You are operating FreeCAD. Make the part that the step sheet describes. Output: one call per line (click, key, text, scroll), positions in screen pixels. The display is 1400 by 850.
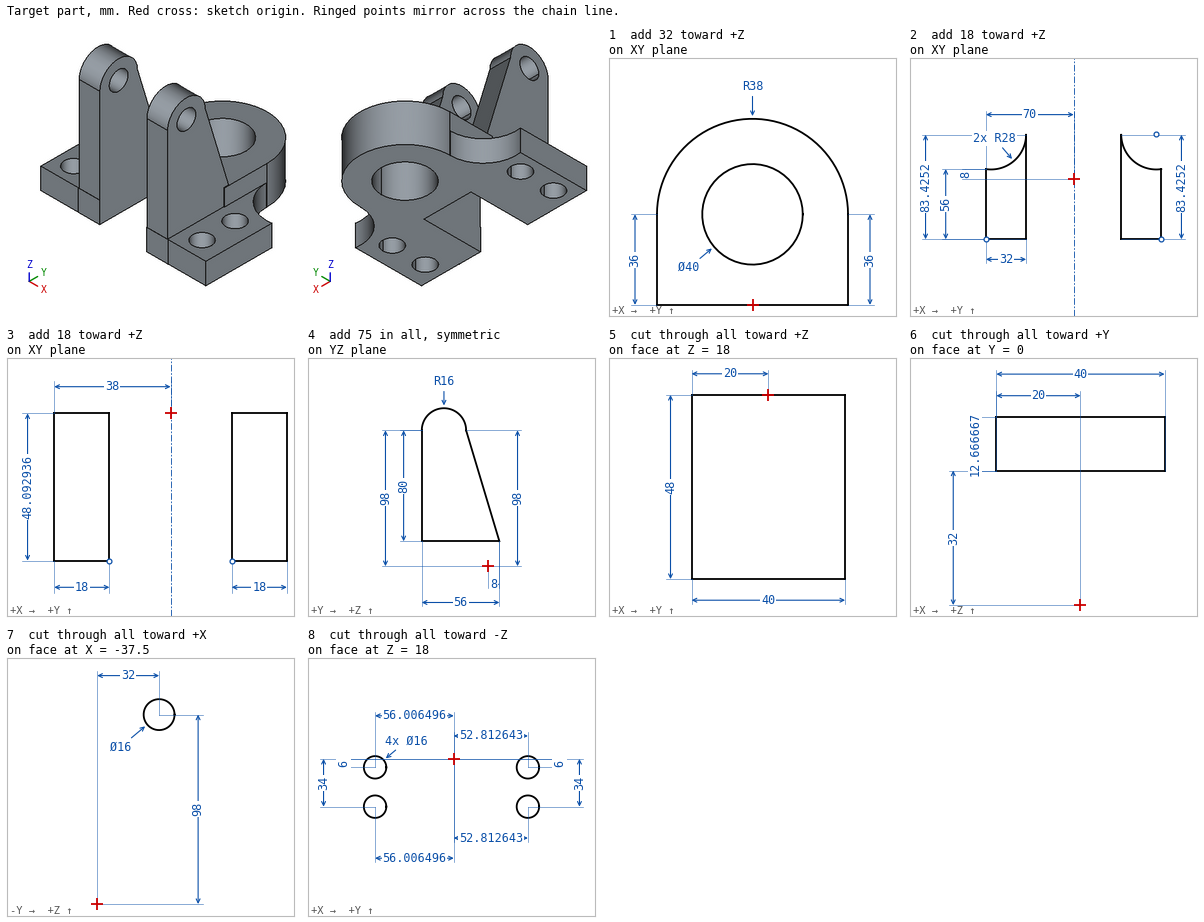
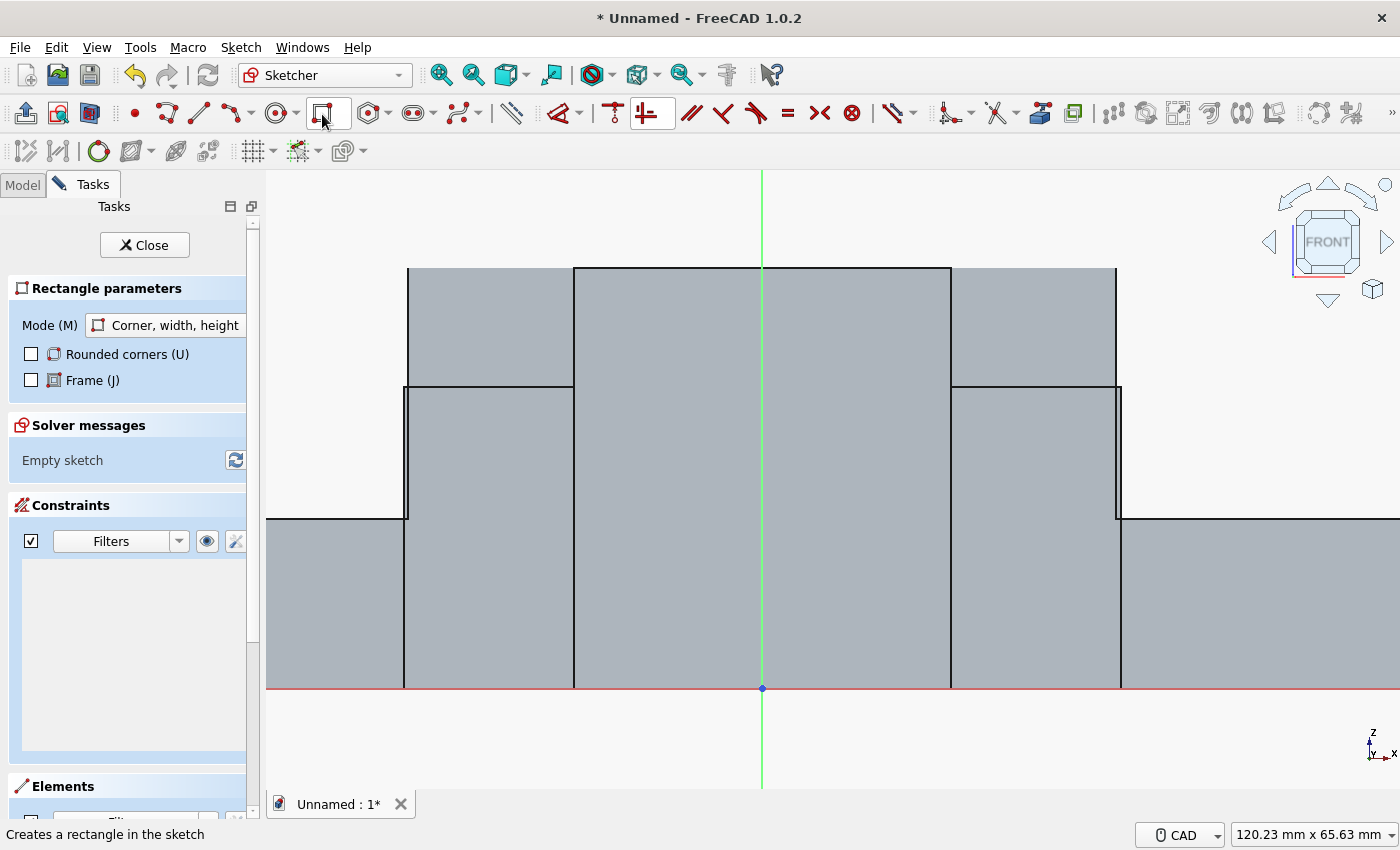
click(574, 268)
click(951, 387)
key(Escape)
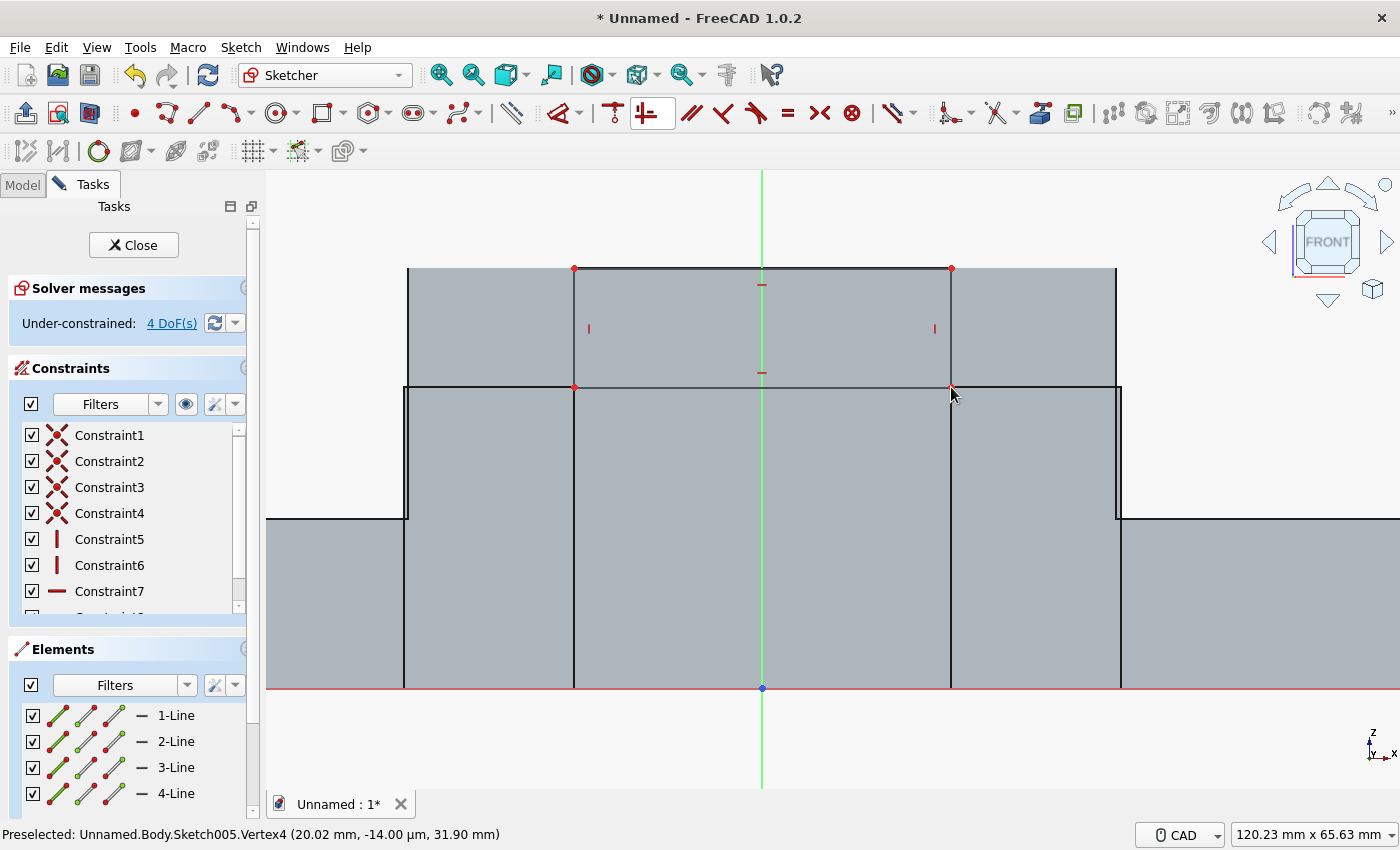
click(558, 114)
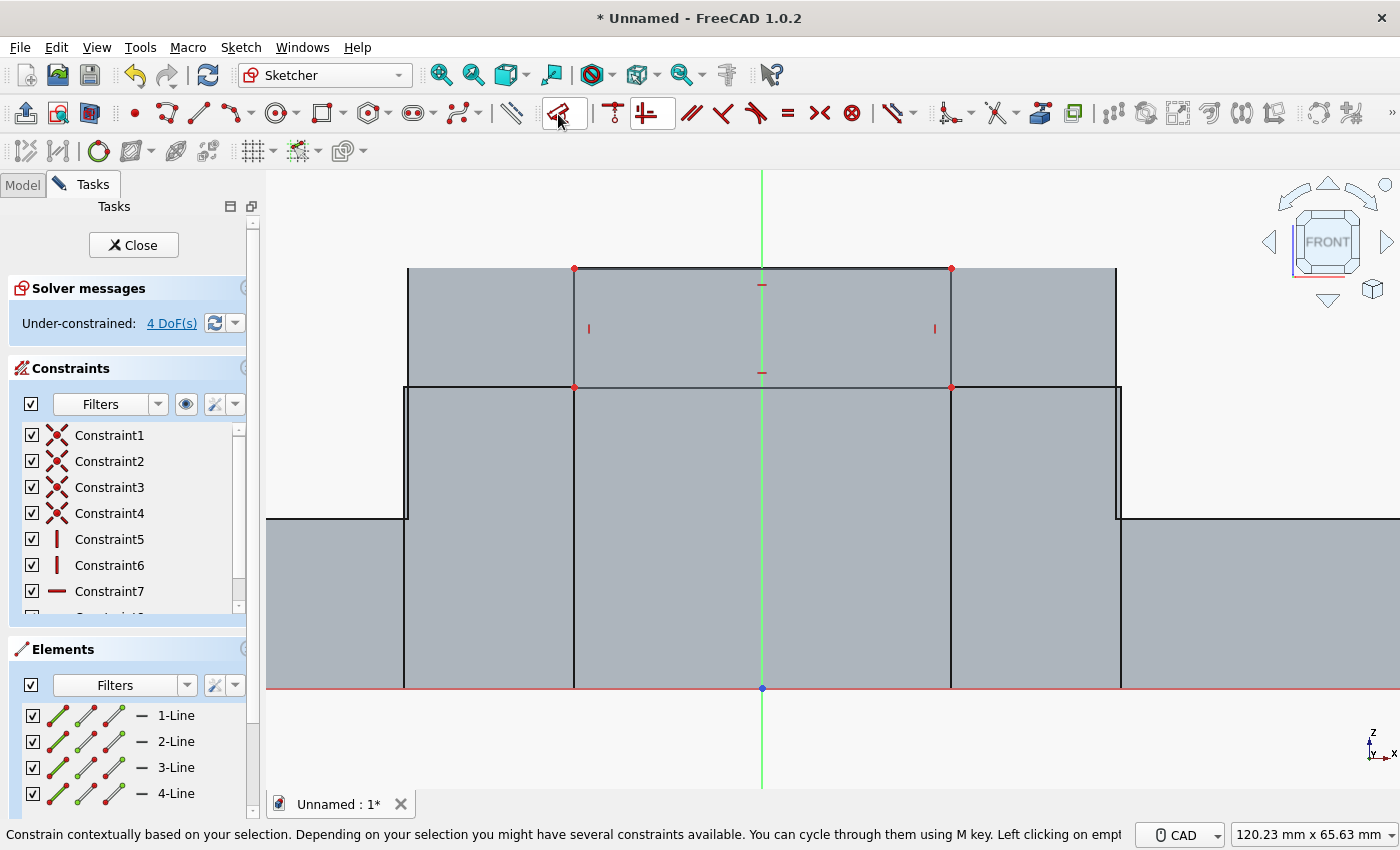
click(687, 388)
click(676, 354)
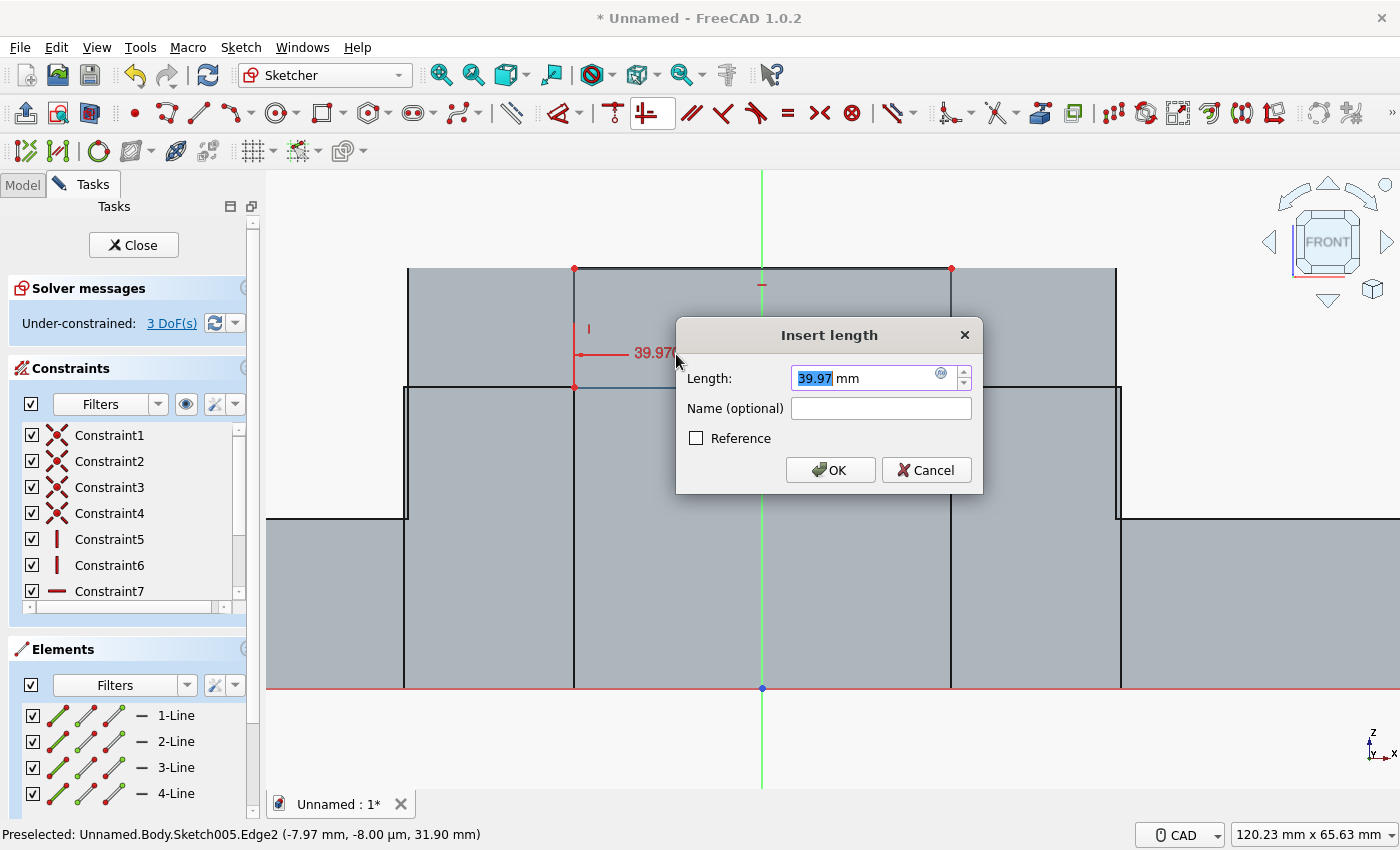
text(40)
key(Return)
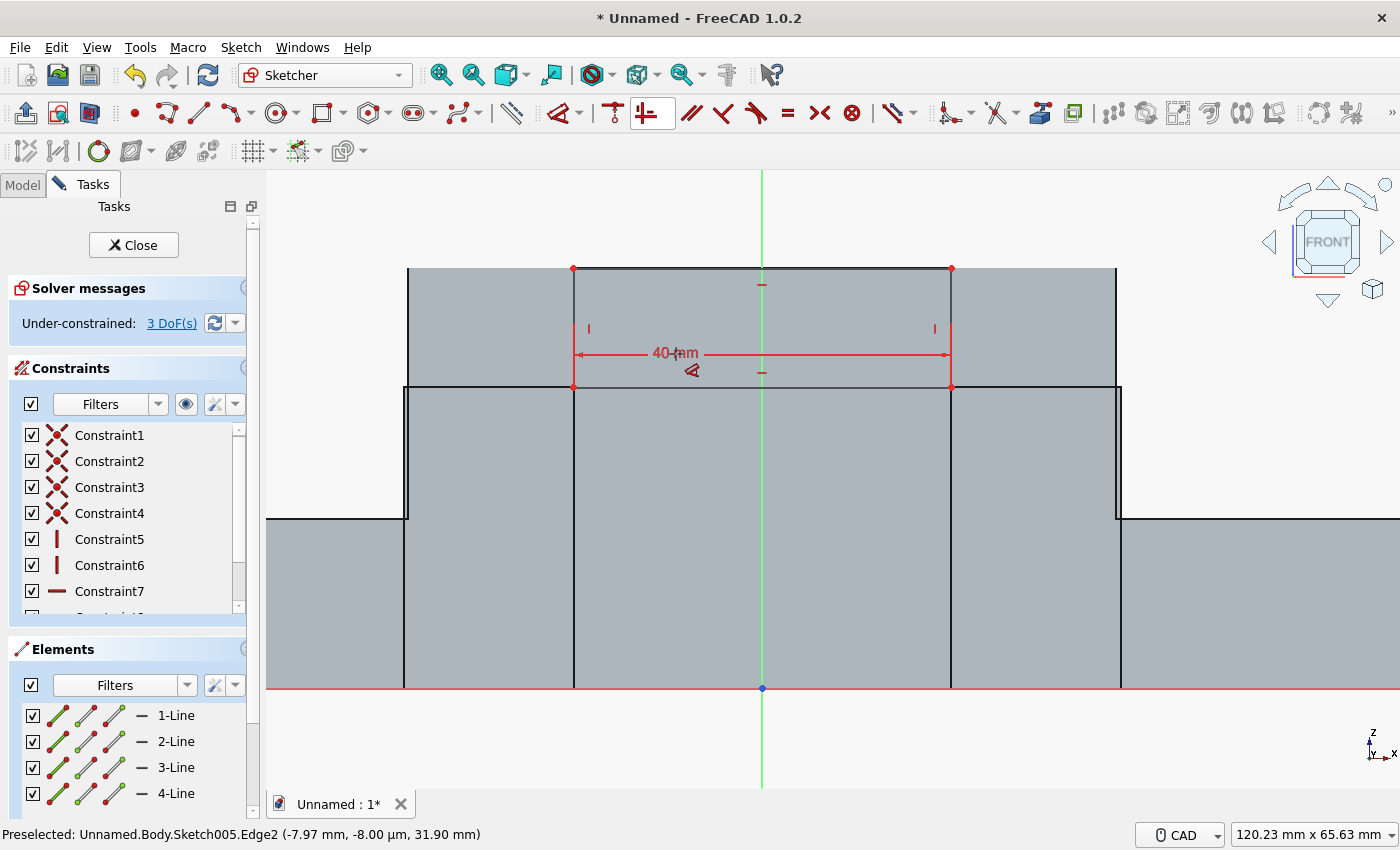
click(574, 269)
click(668, 723)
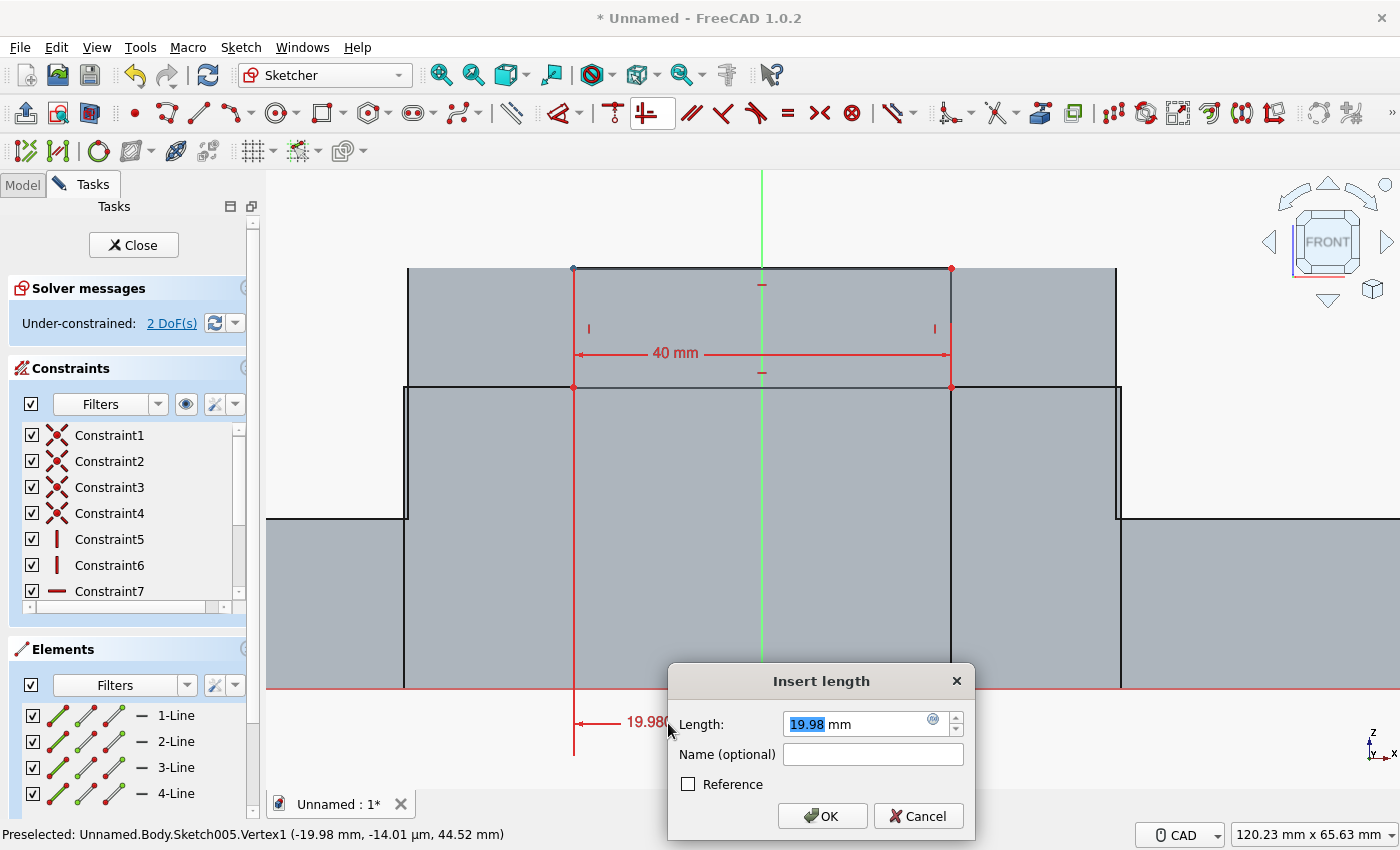
text(20)
key(Return)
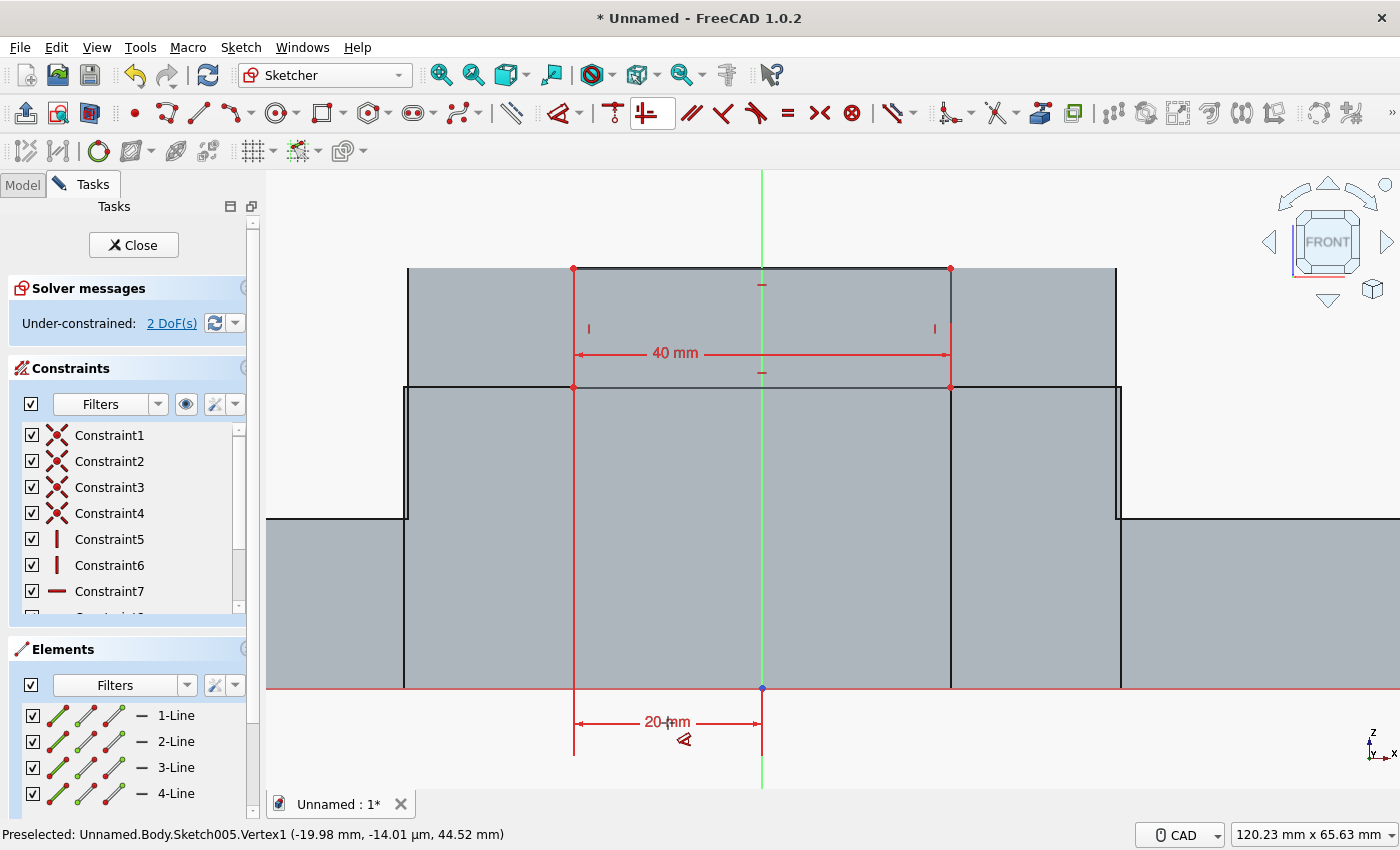
click(574, 388)
click(540, 538)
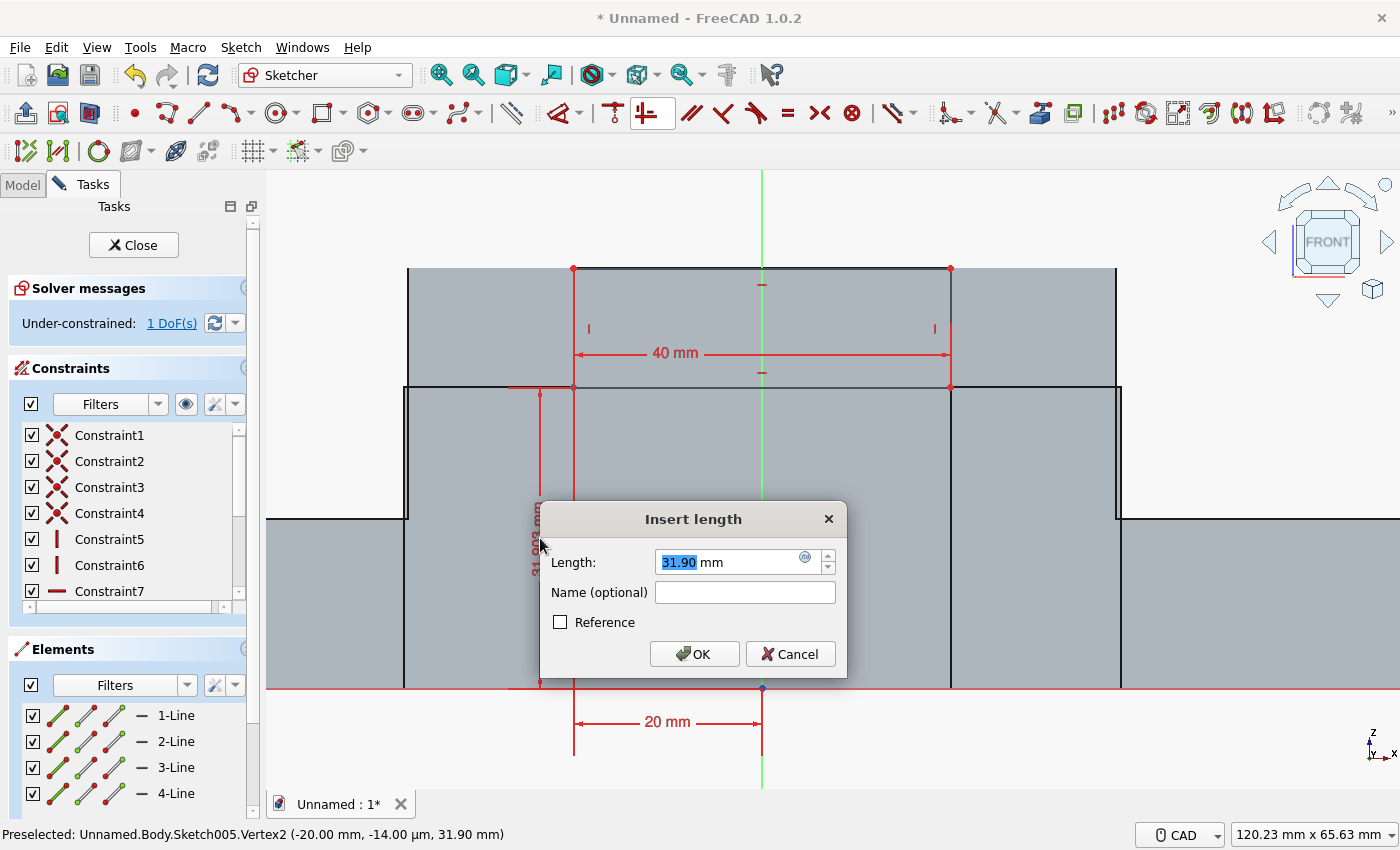
text(32)
key(Return)